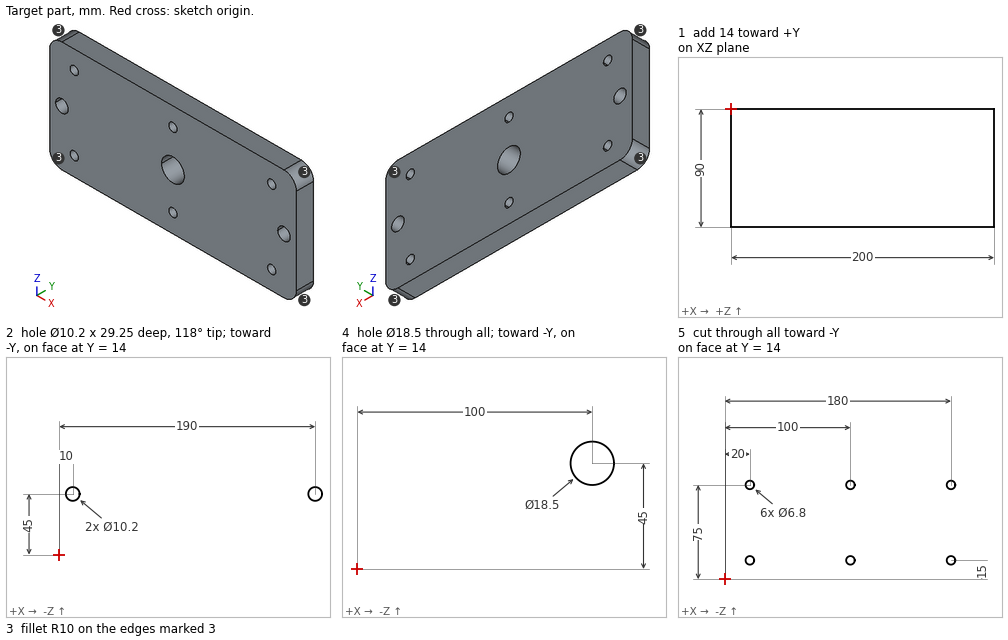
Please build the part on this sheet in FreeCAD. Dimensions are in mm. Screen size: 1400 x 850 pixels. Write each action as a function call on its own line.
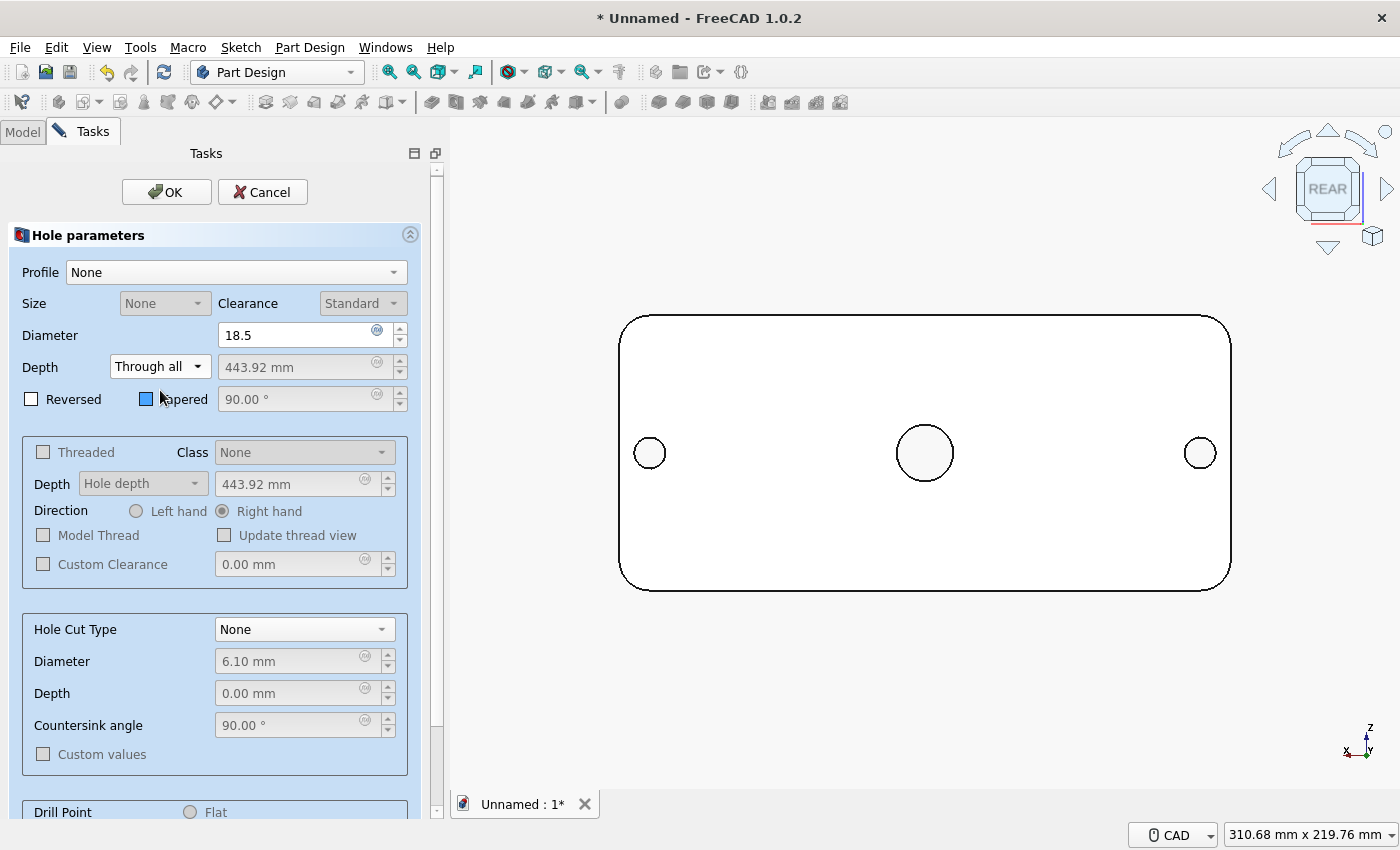
click(167, 192)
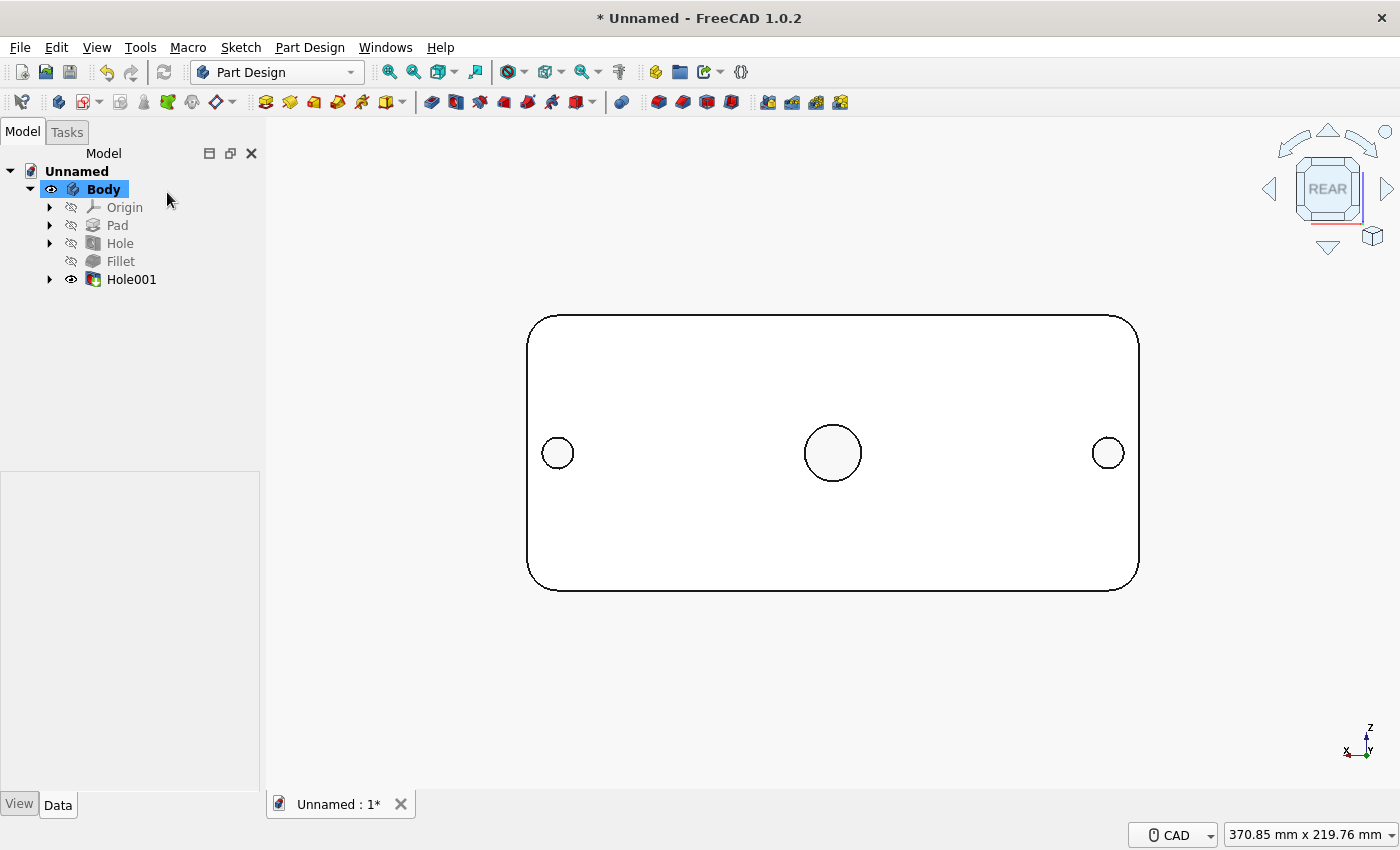
click(1008, 413)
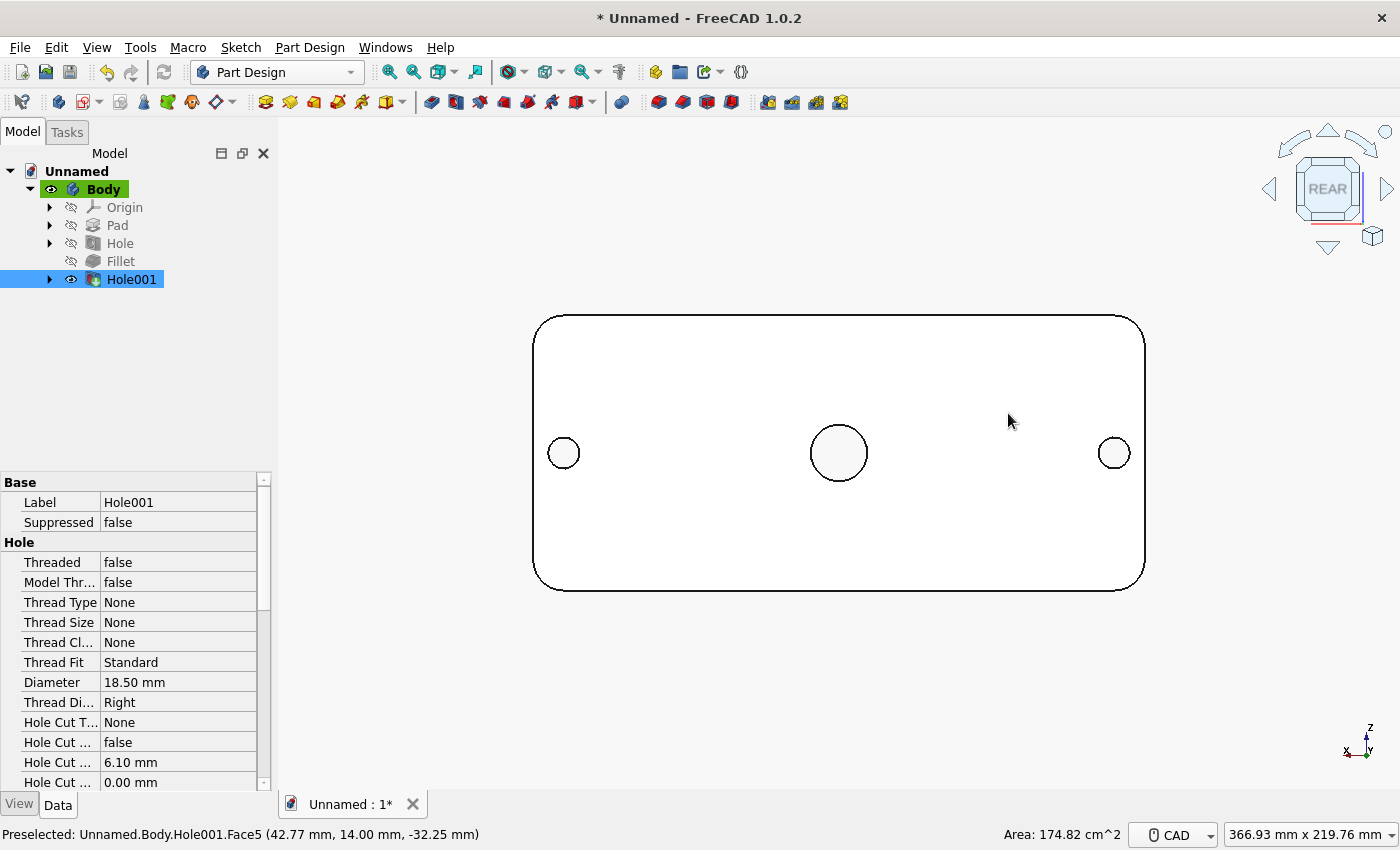
click(84, 102)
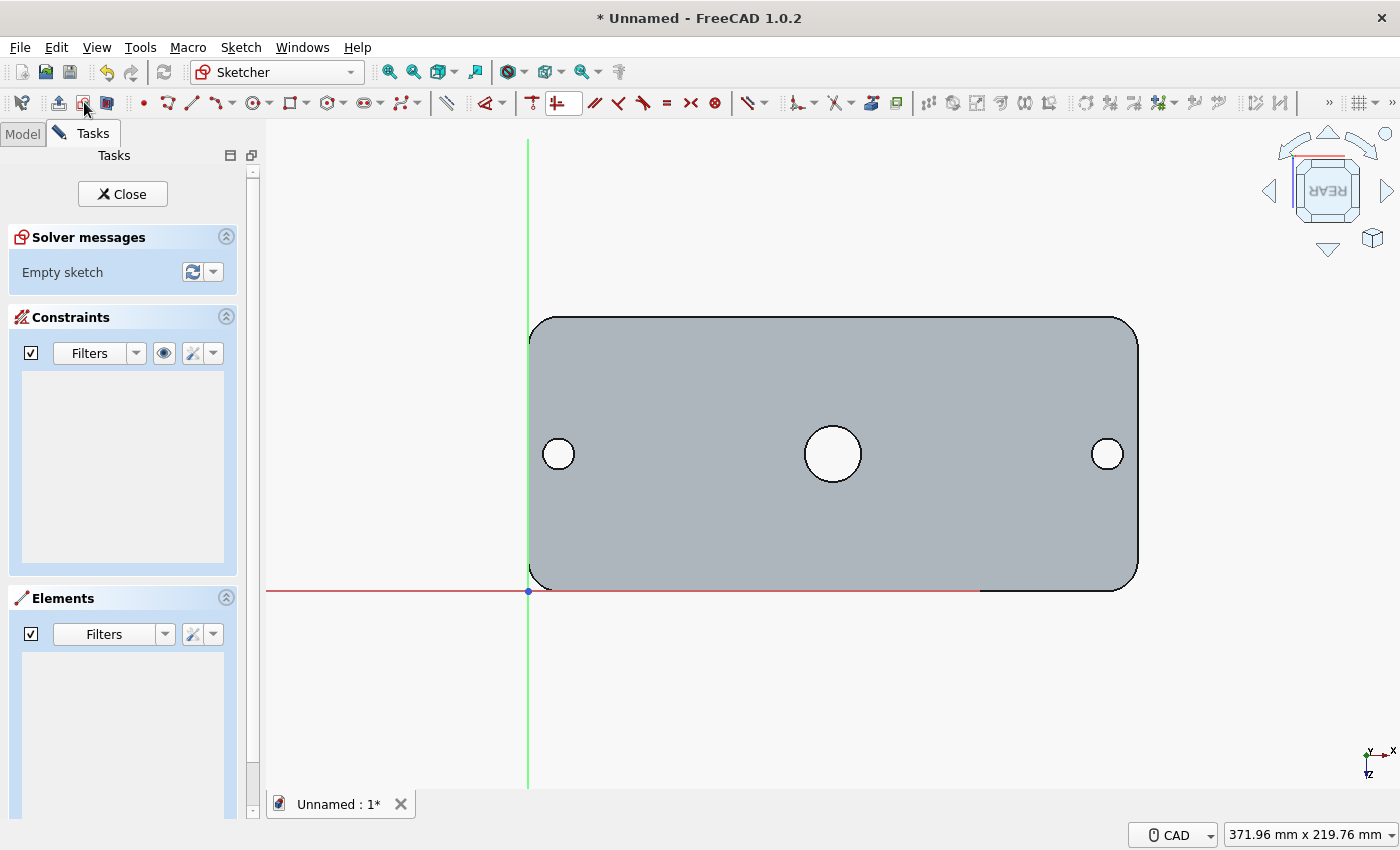
click(254, 104)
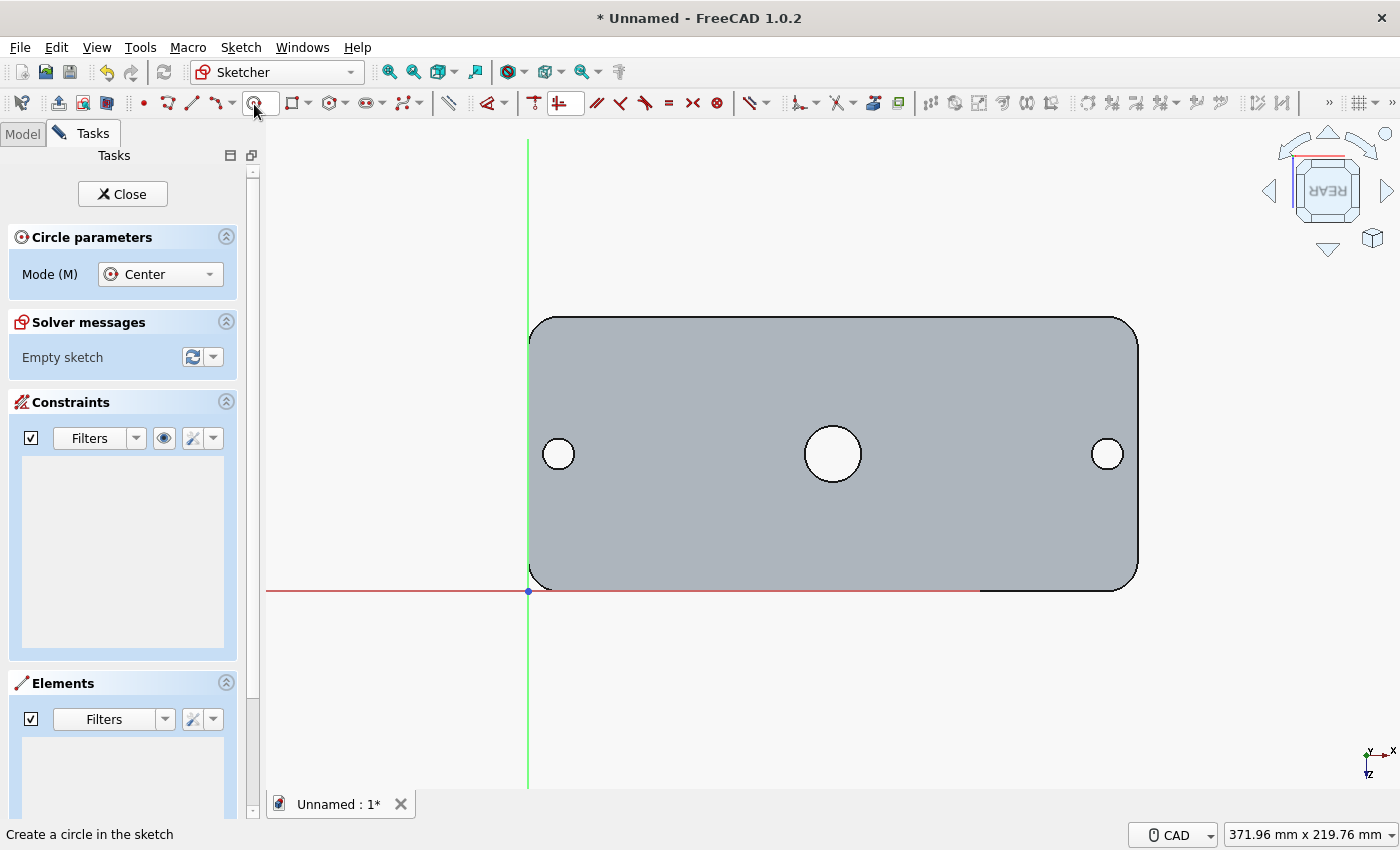
scroll(589, 363, up, 4)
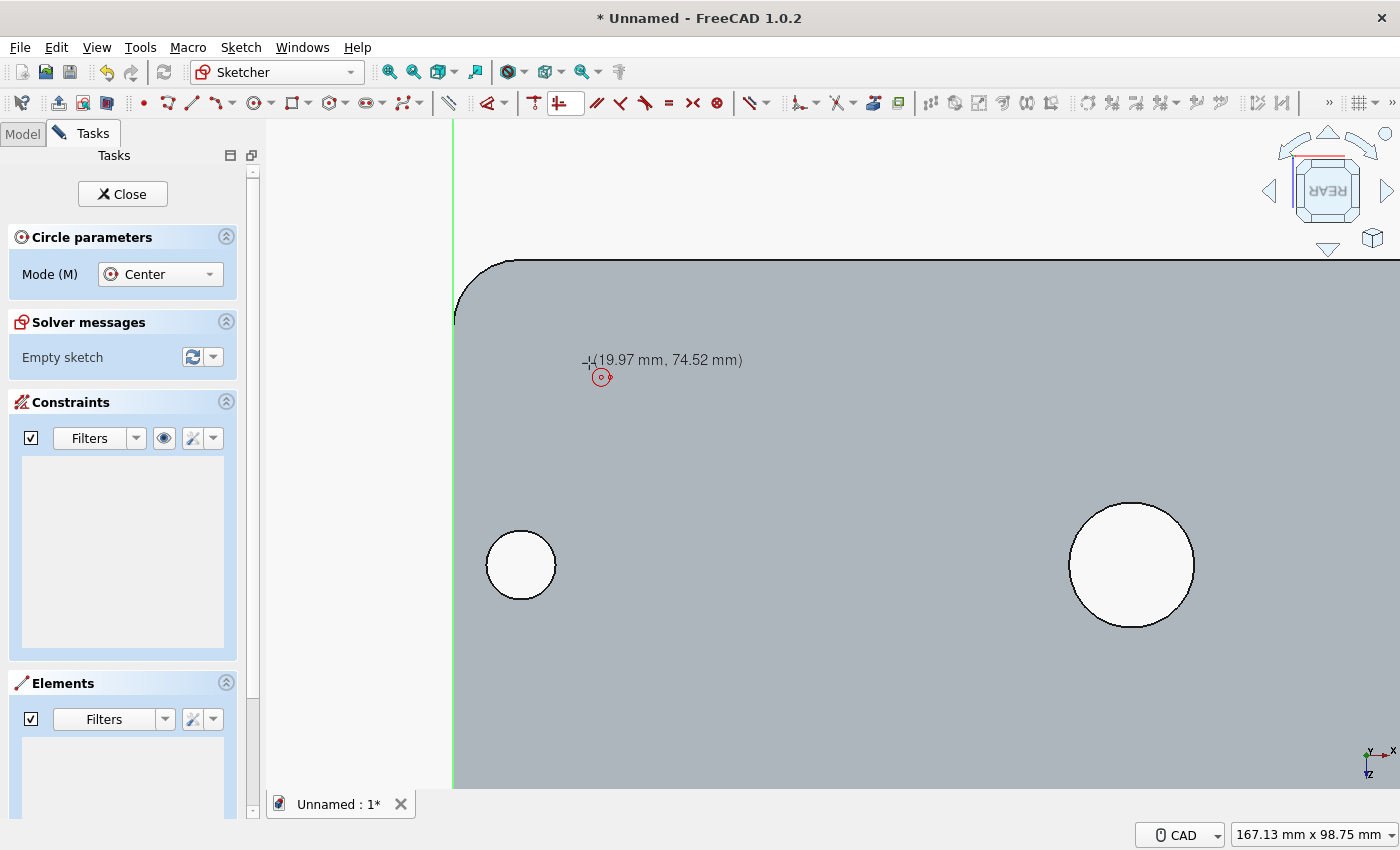
click(589, 362)
click(605, 345)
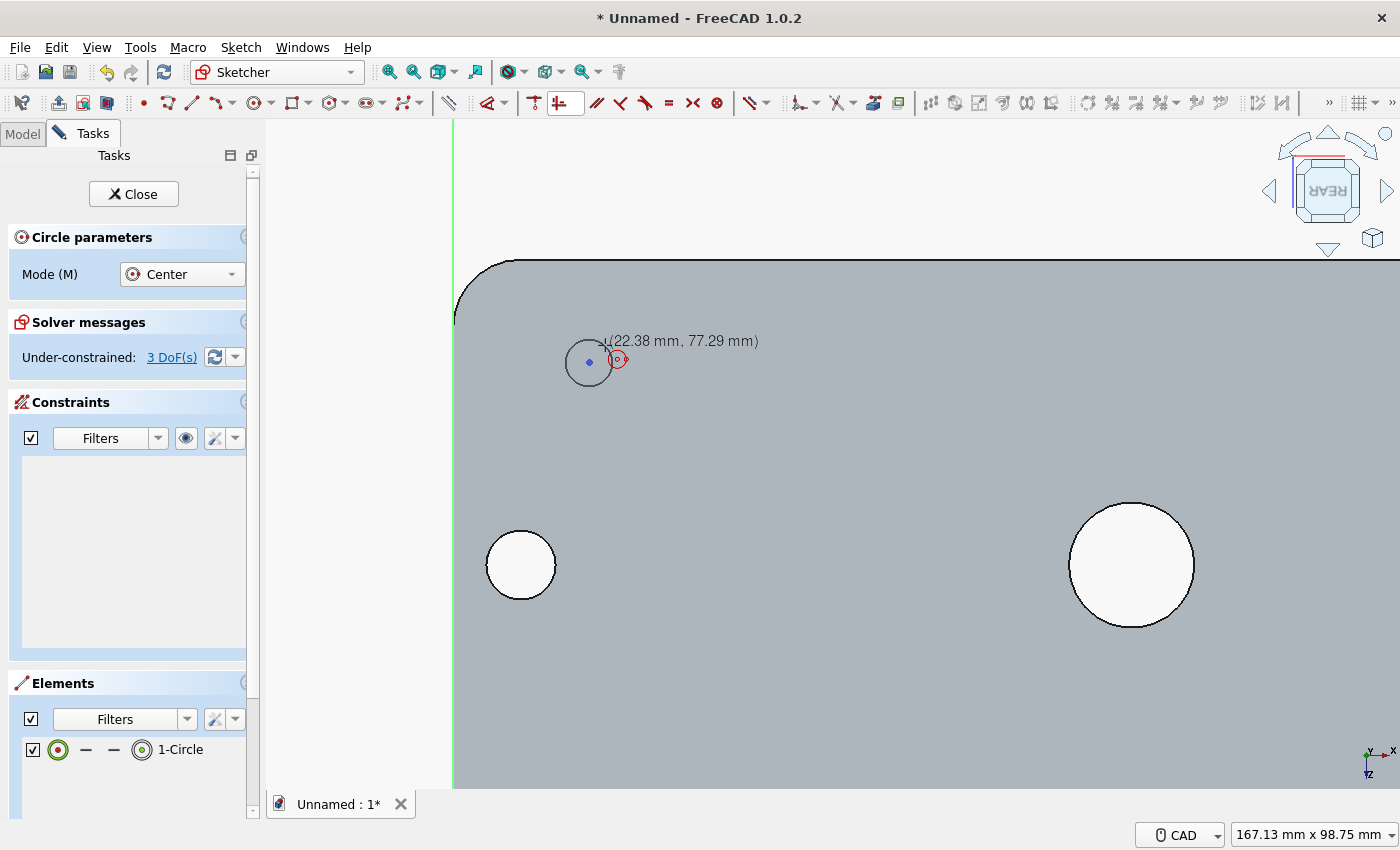
click(1132, 362)
click(1148, 345)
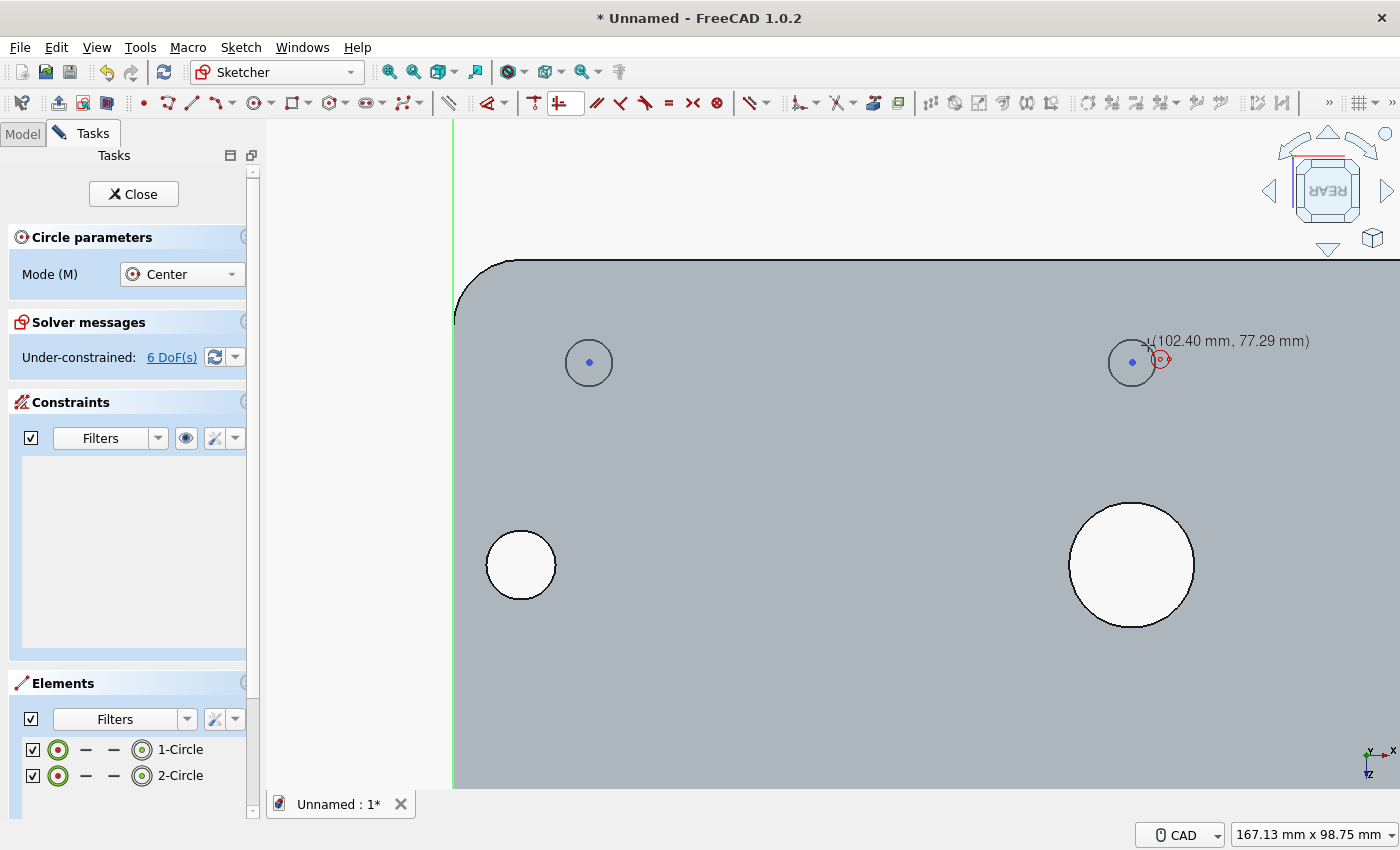
scroll(386, 271, down, 3)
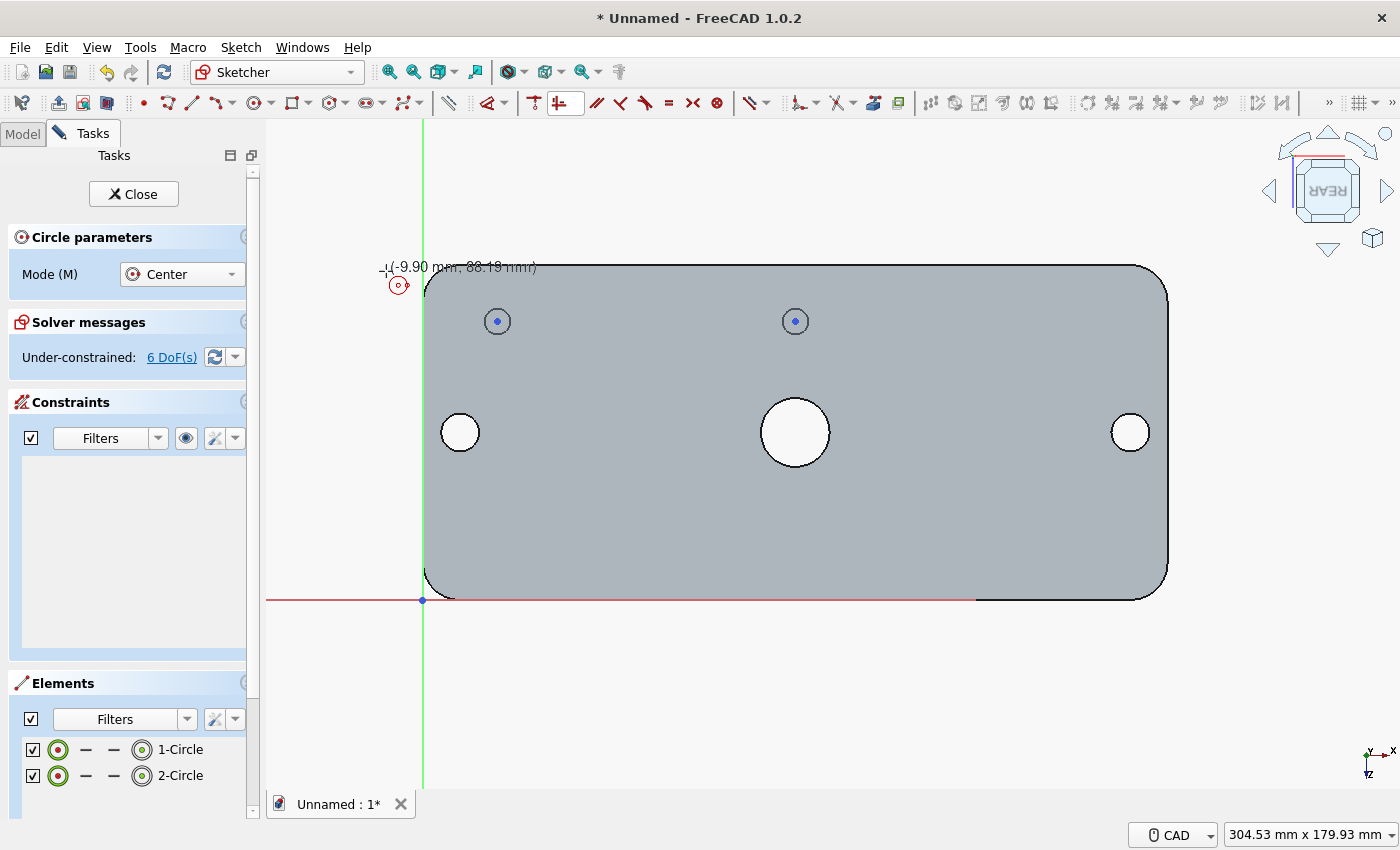
scroll(1093, 321, up, 3)